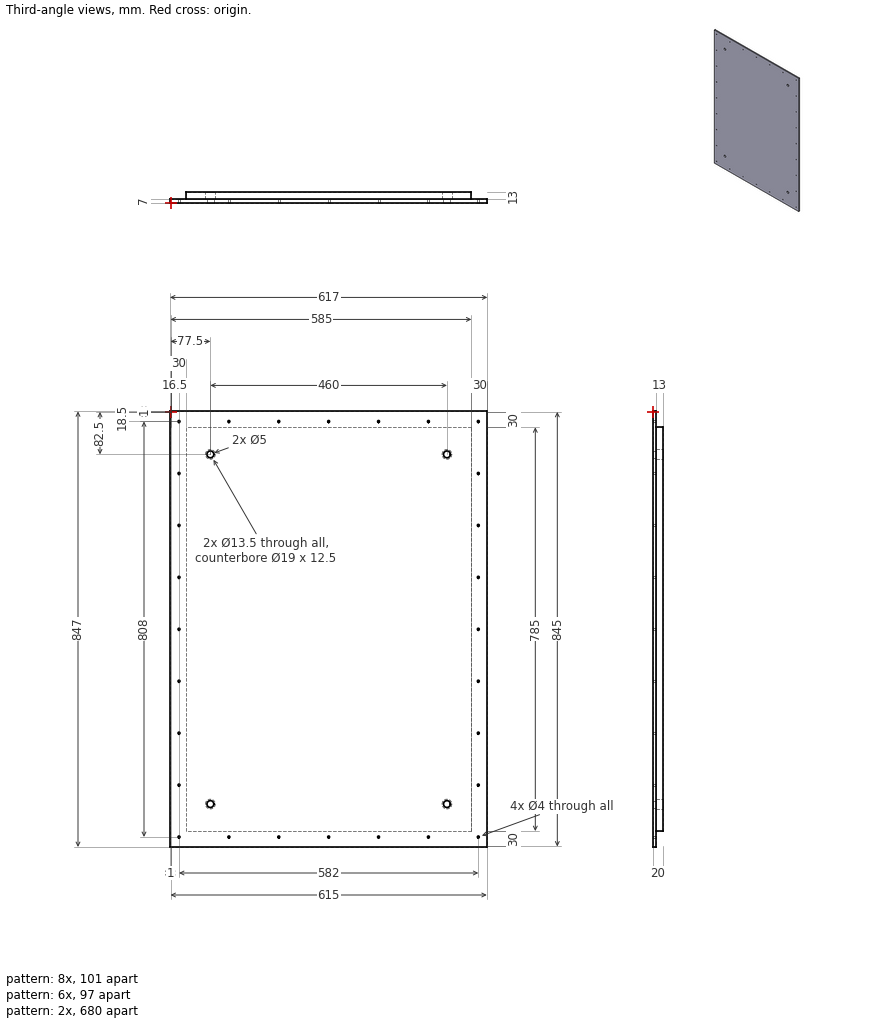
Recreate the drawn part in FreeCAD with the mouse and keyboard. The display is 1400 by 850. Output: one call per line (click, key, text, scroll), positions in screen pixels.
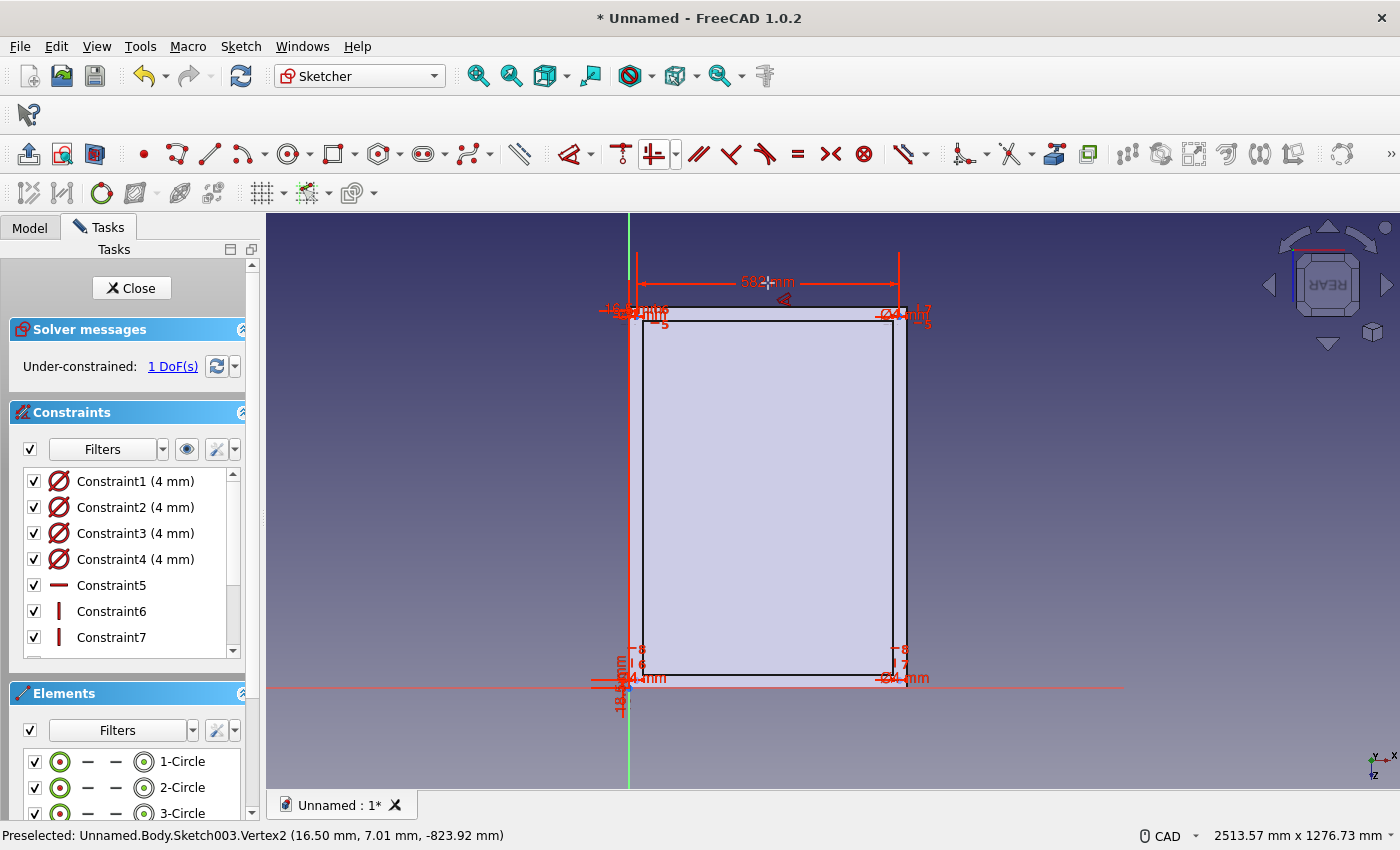
click(637, 317)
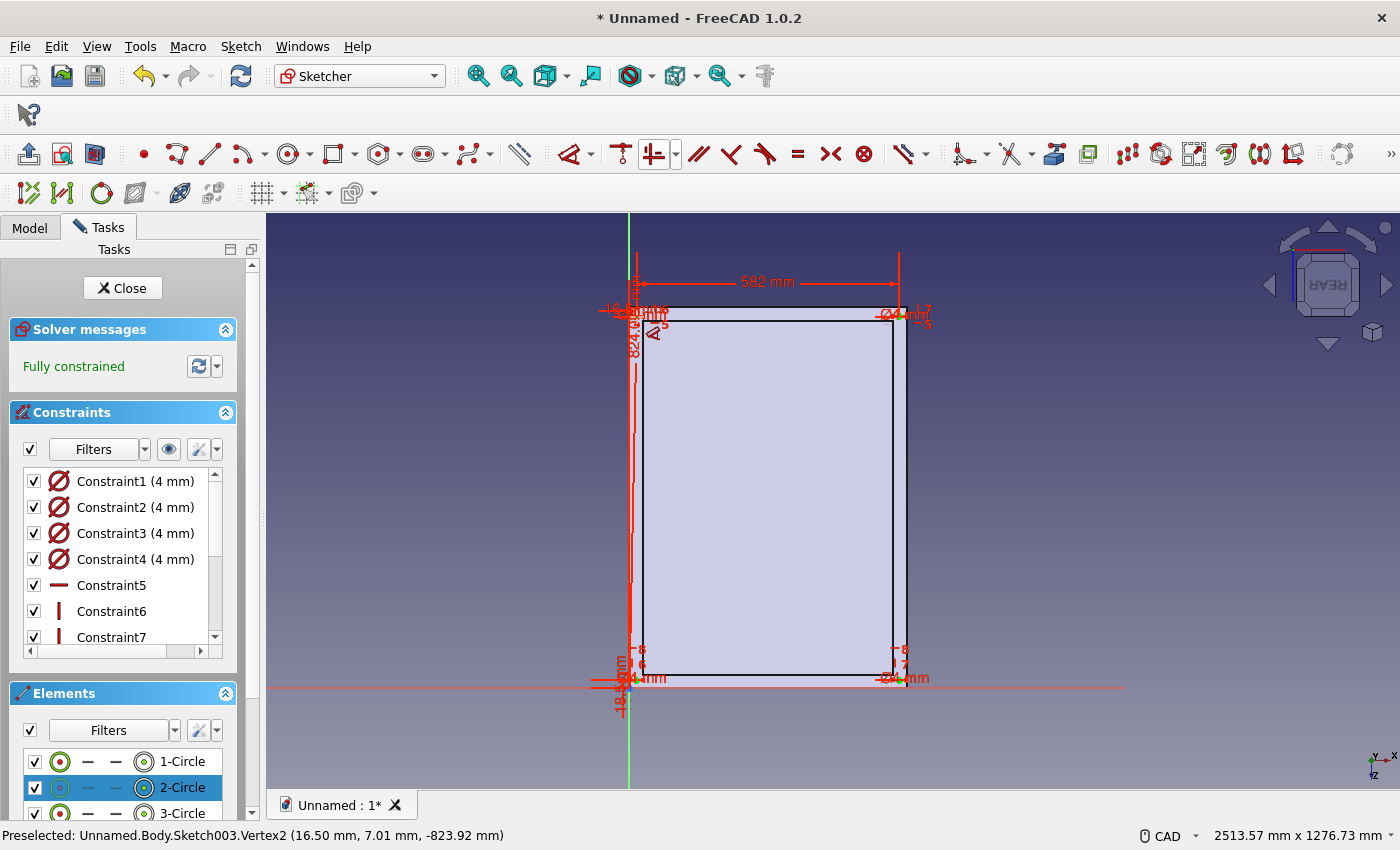
click(637, 680)
click(603, 498)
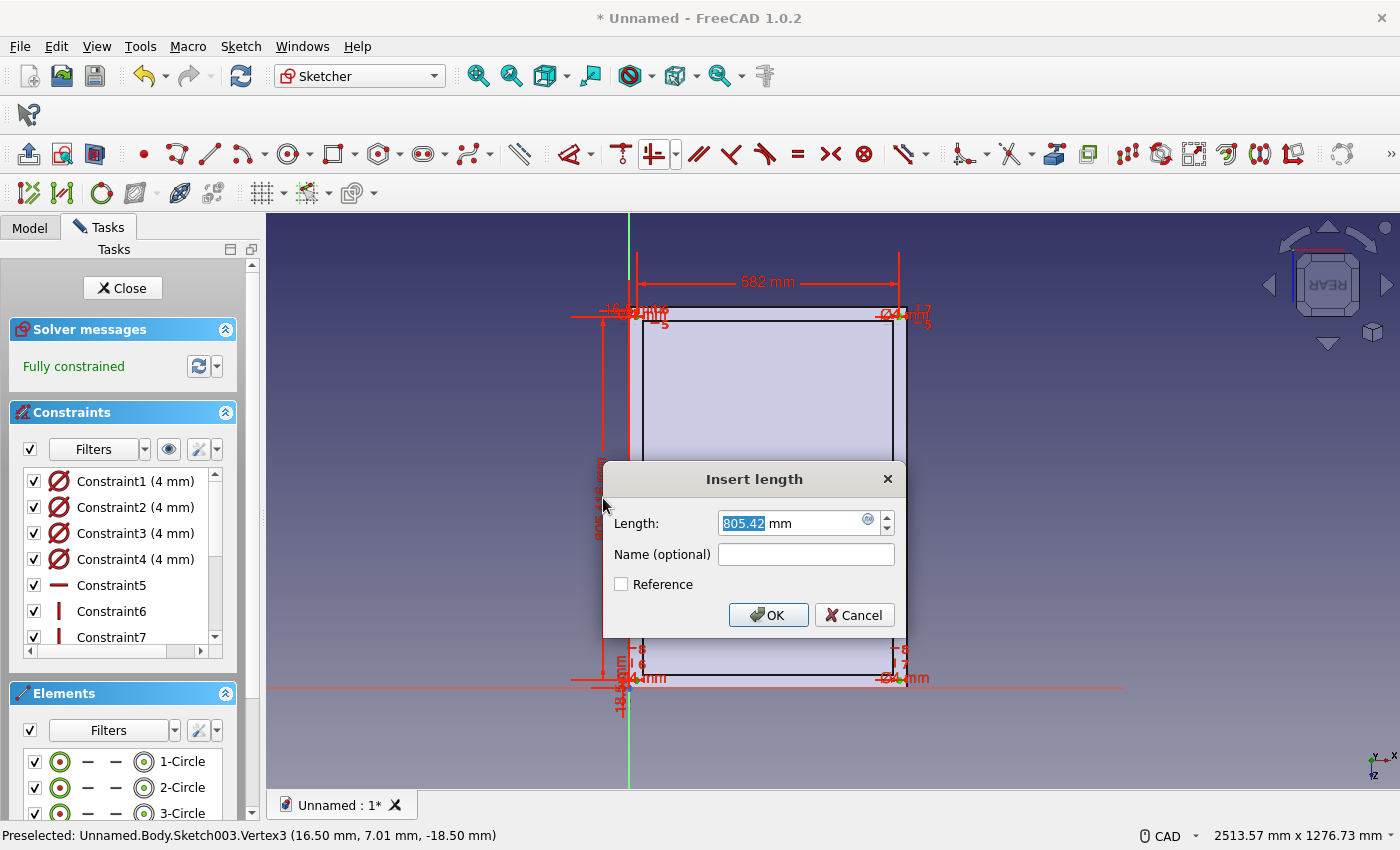
text(808)
key(Return)
key(Escape)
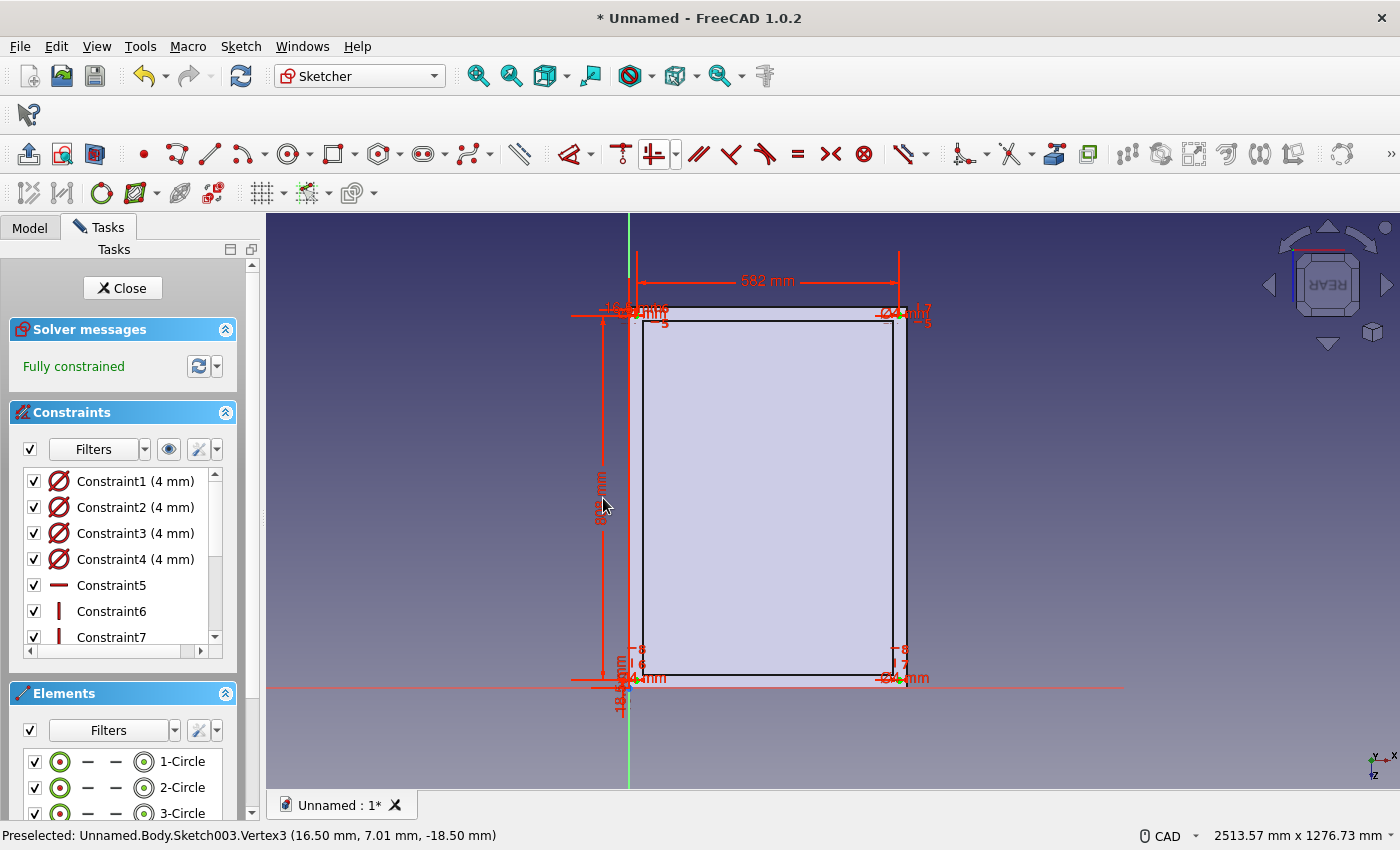
click(123, 288)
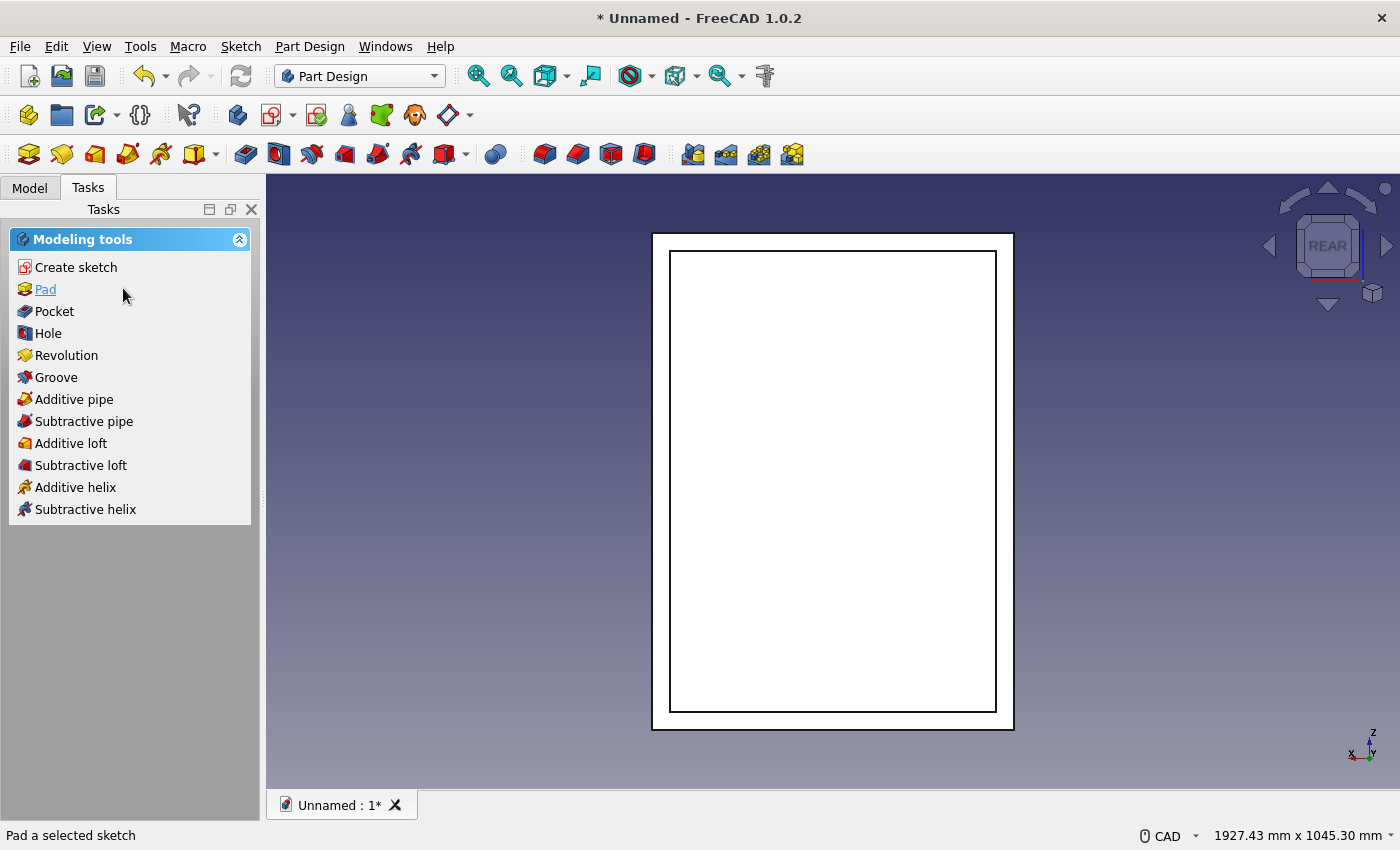
click(279, 154)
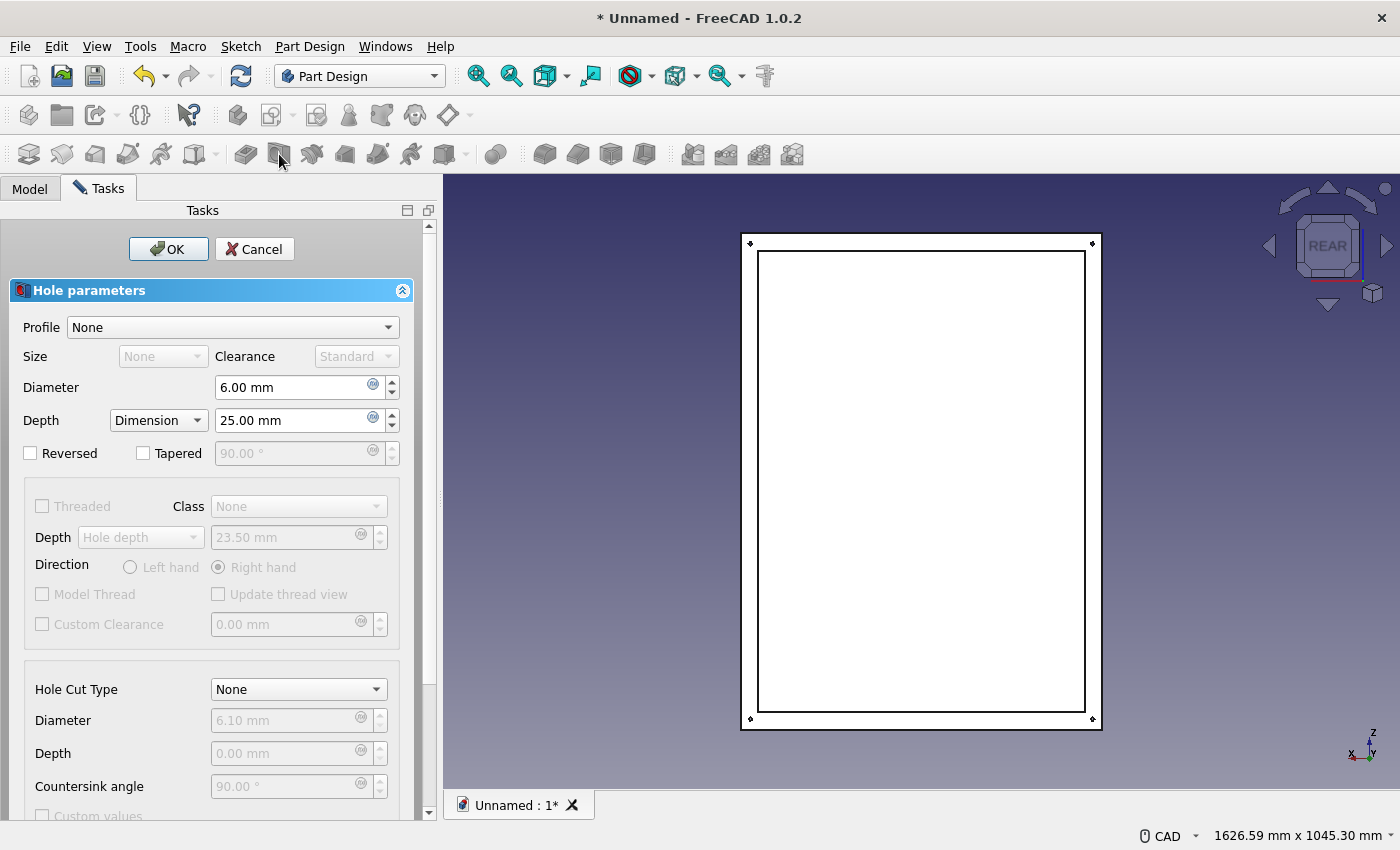
triple_click(300, 388)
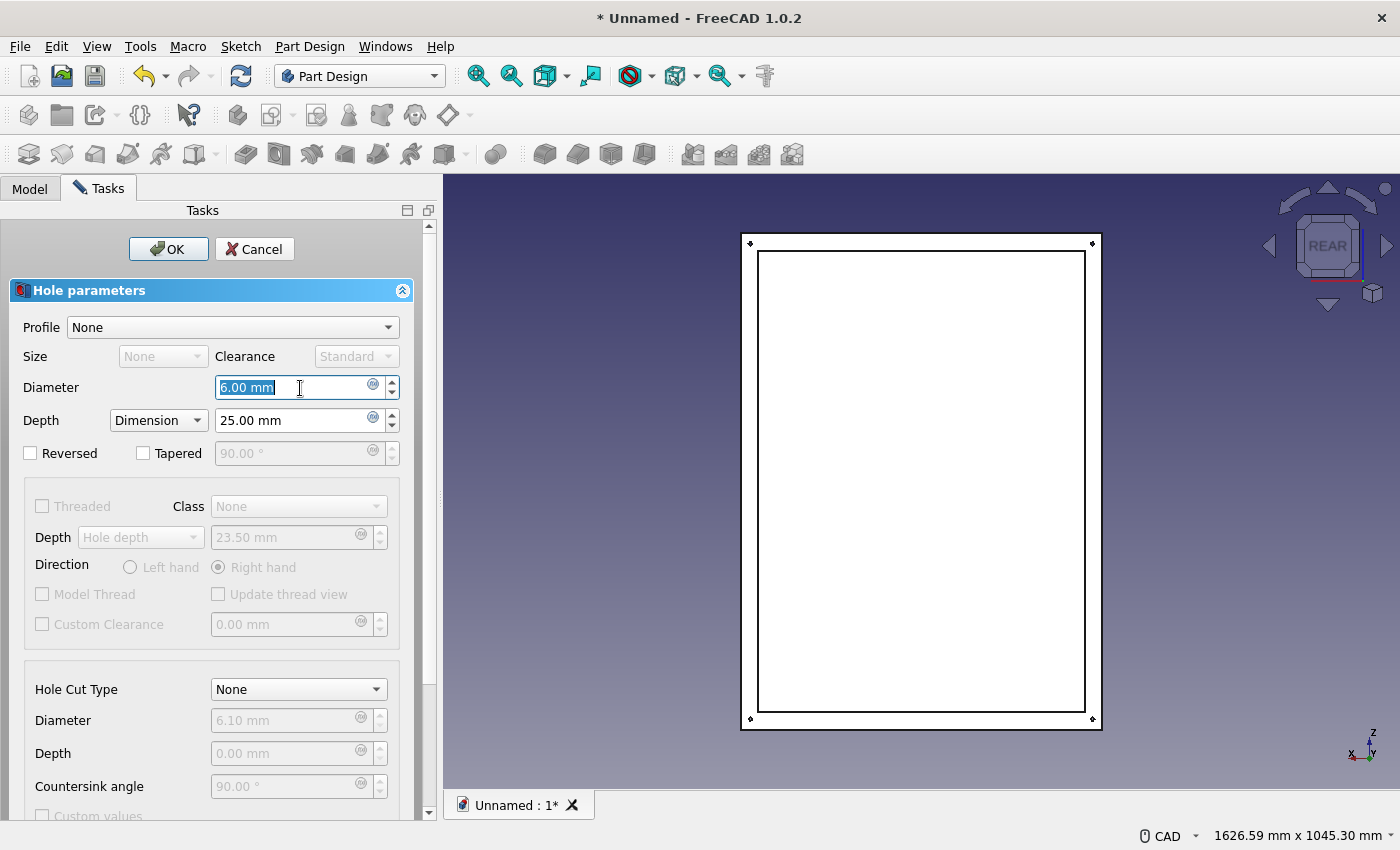
text(4)
key(Tab)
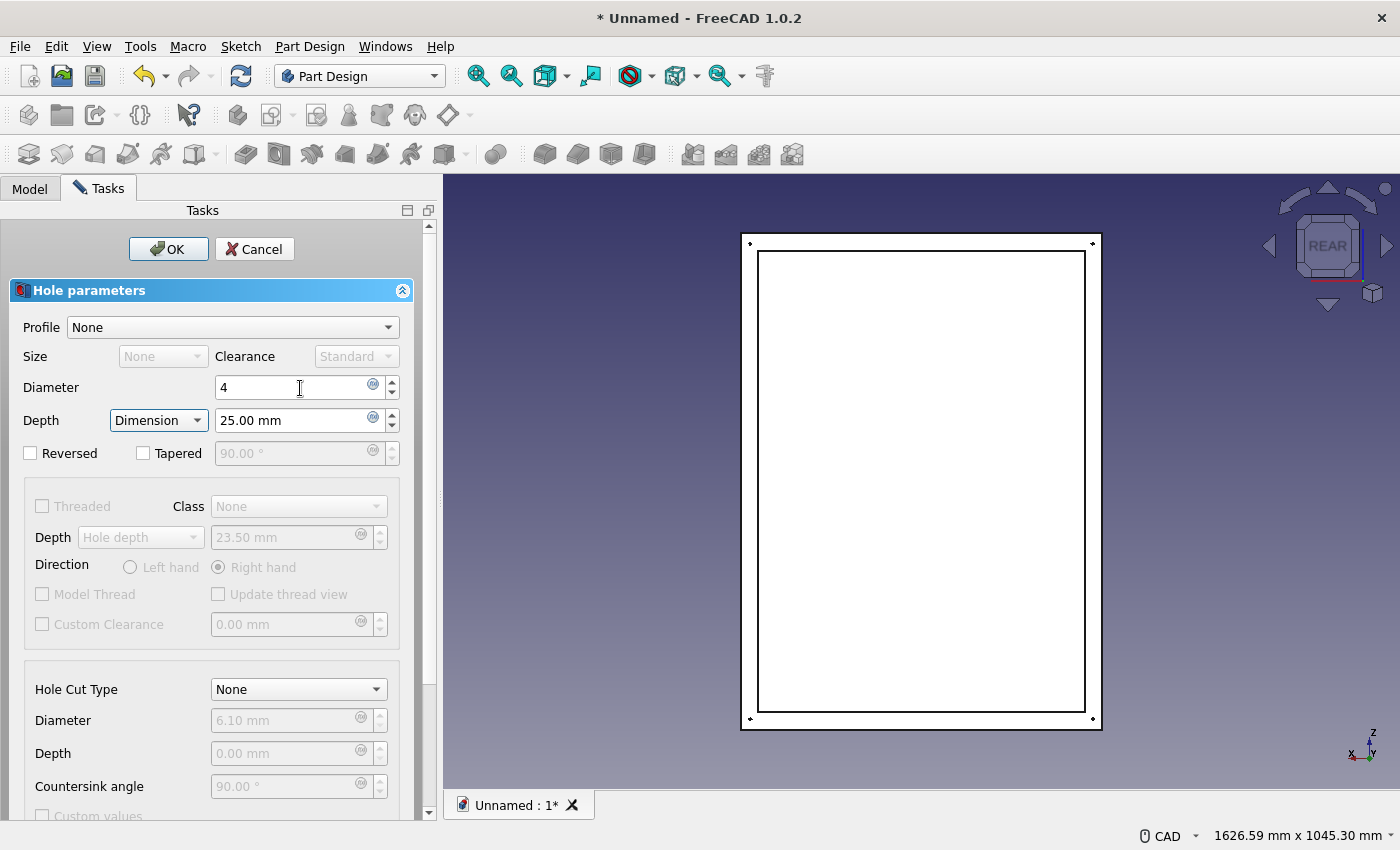
click(160, 420)